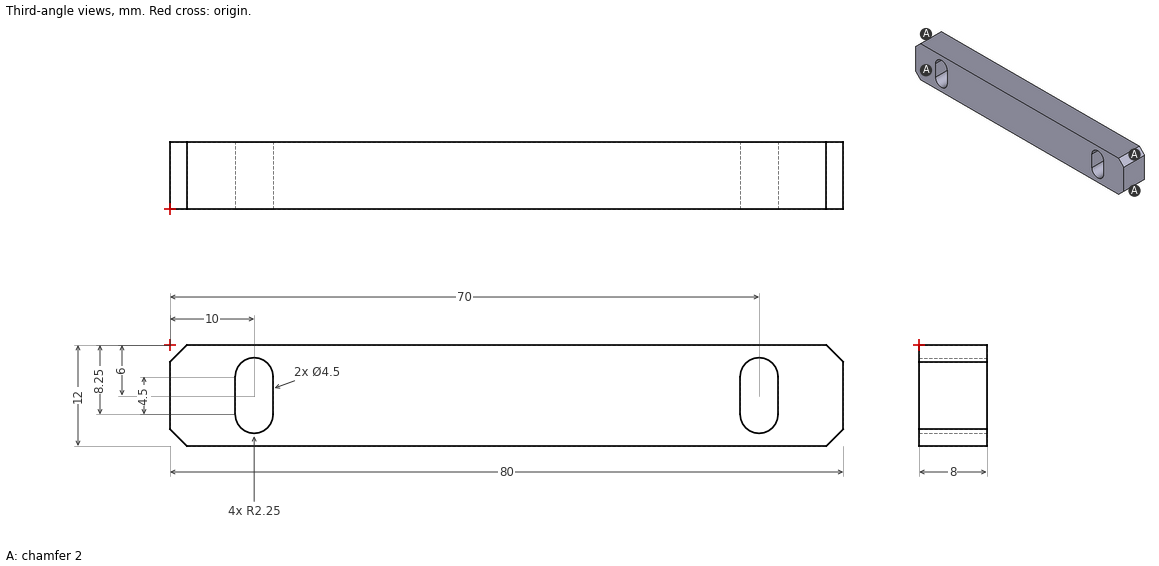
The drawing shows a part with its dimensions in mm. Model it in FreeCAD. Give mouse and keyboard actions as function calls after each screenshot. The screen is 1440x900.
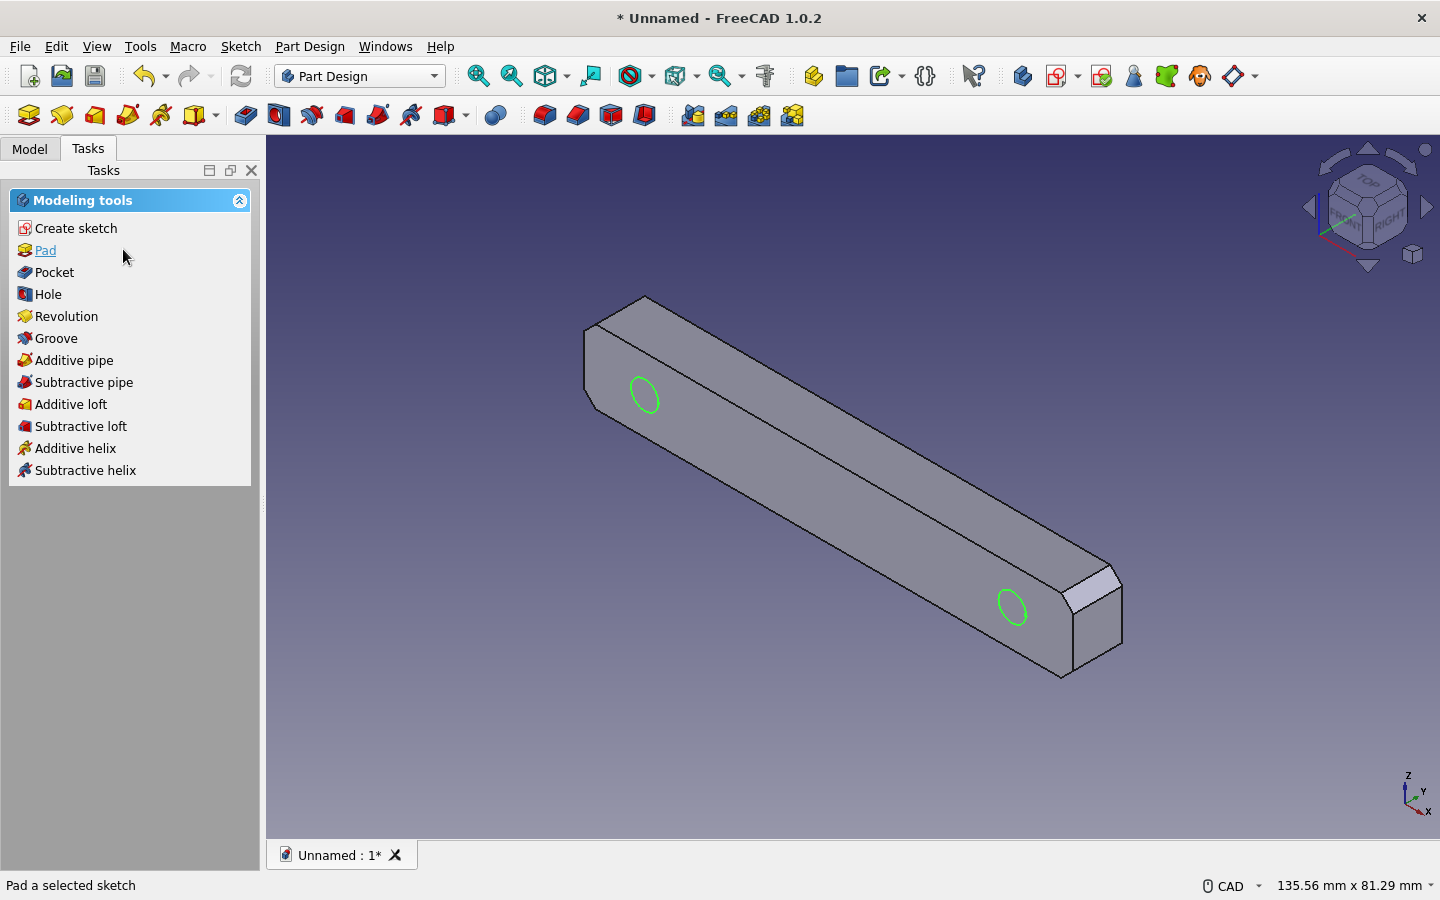
click(246, 116)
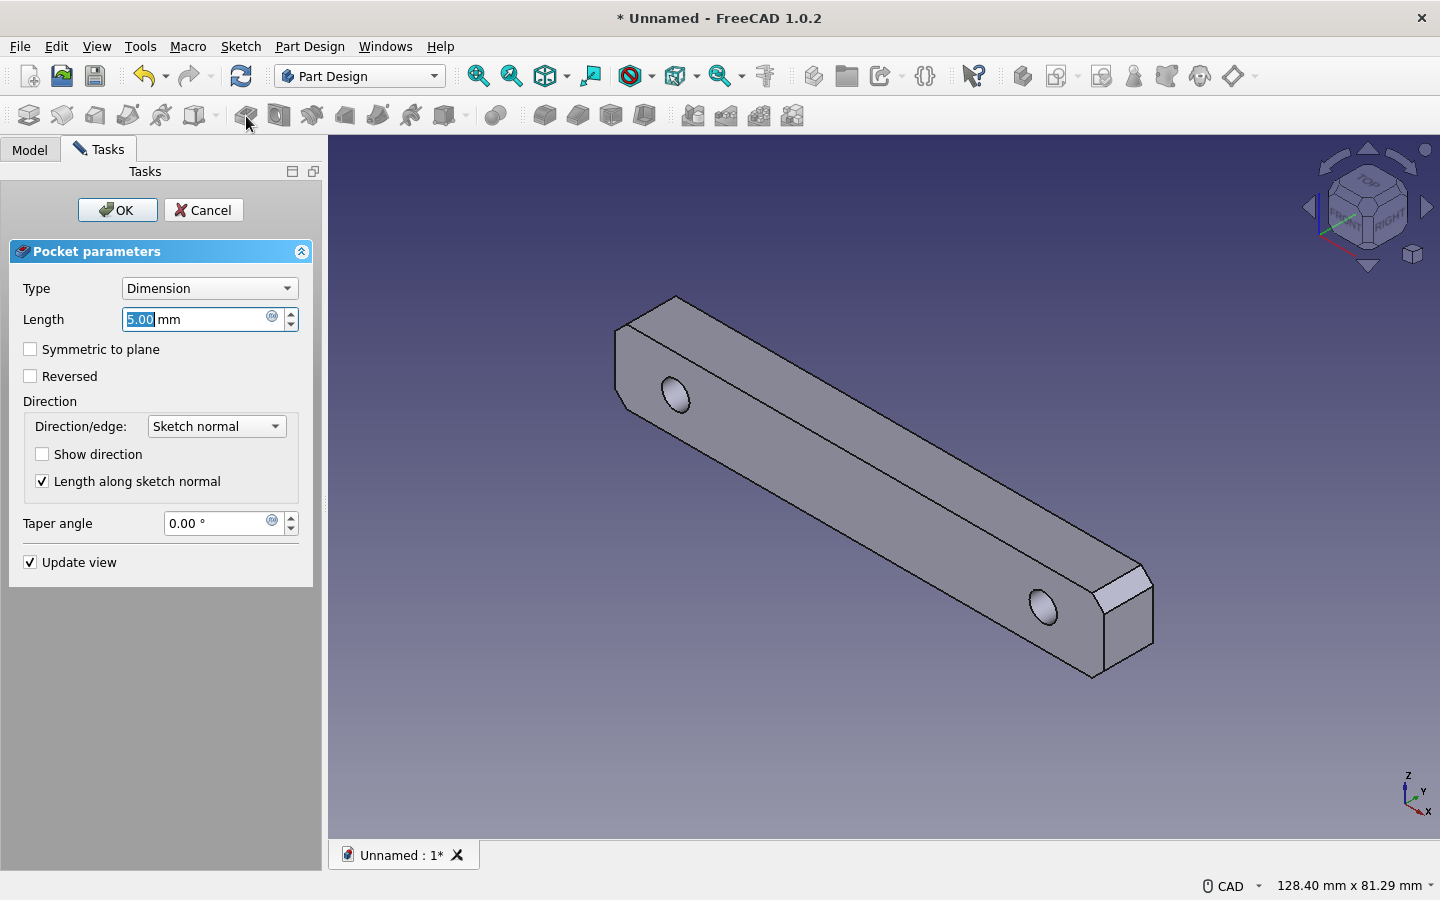
text(10)
key(Tab)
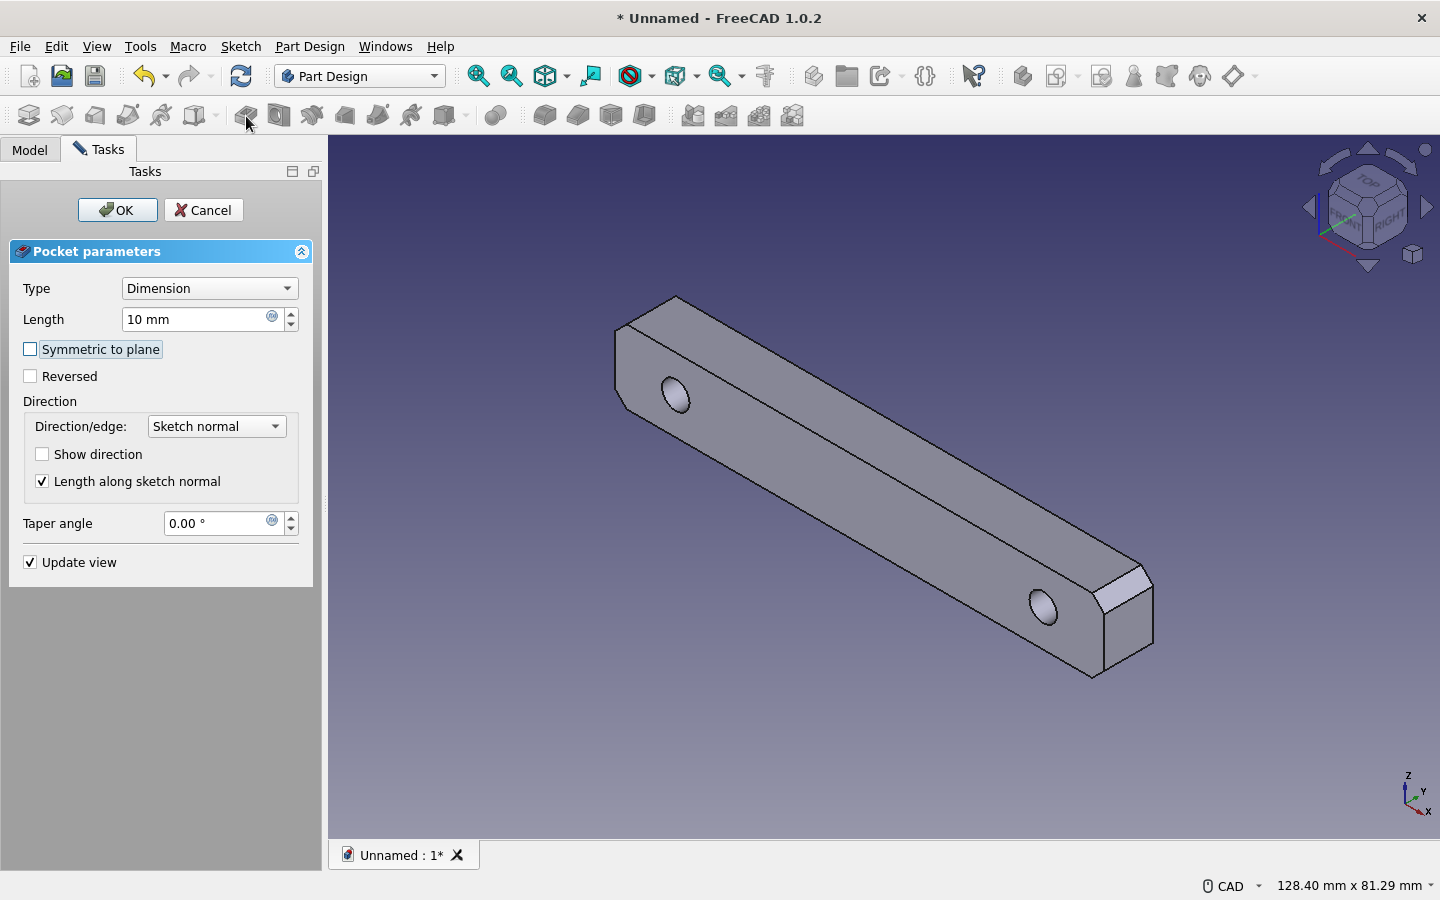
click(118, 210)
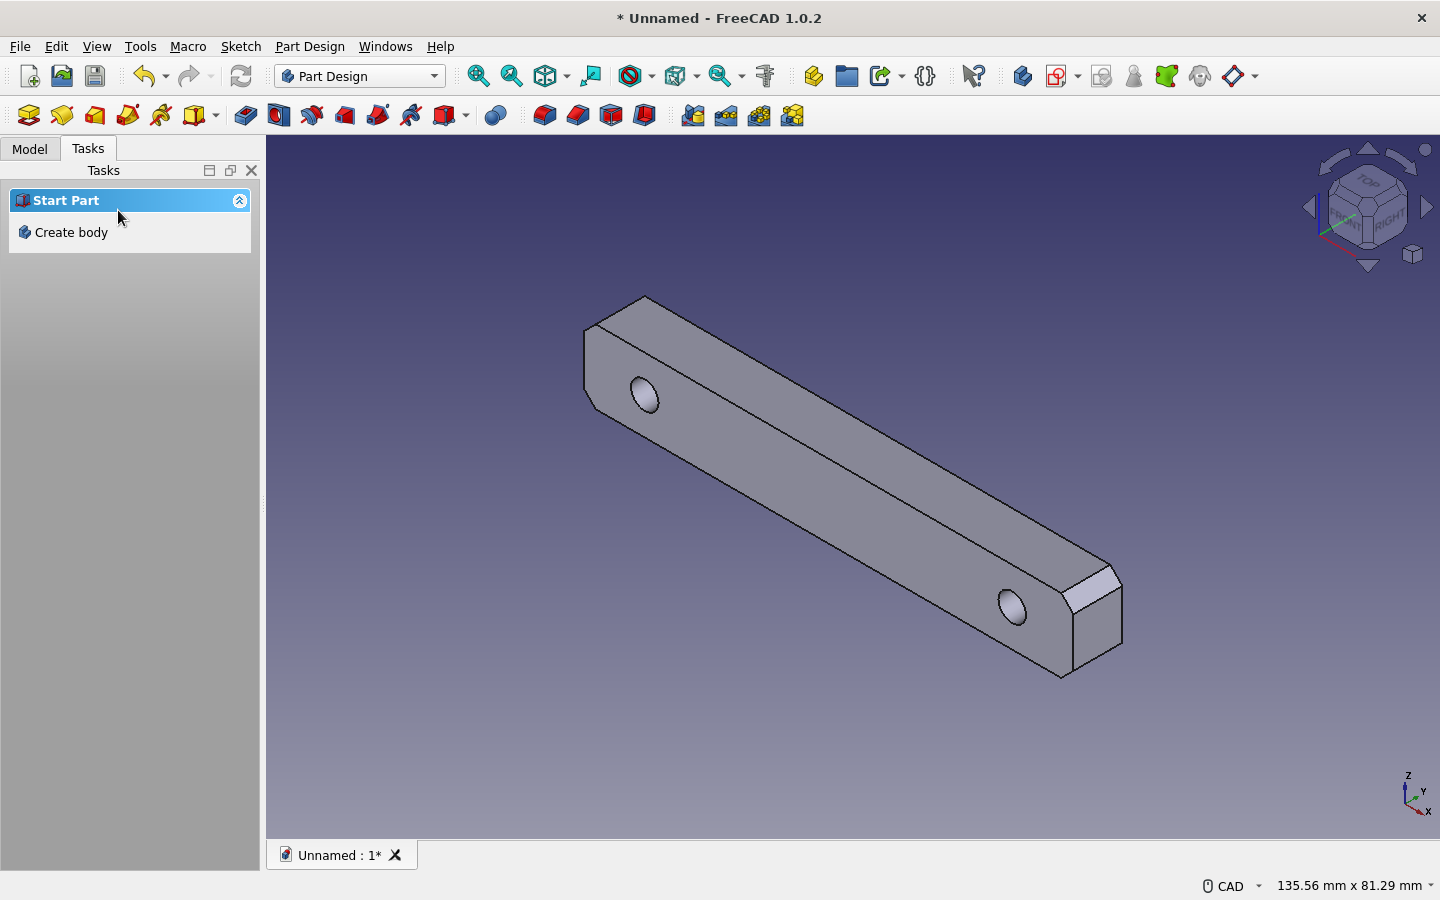
click(1056, 76)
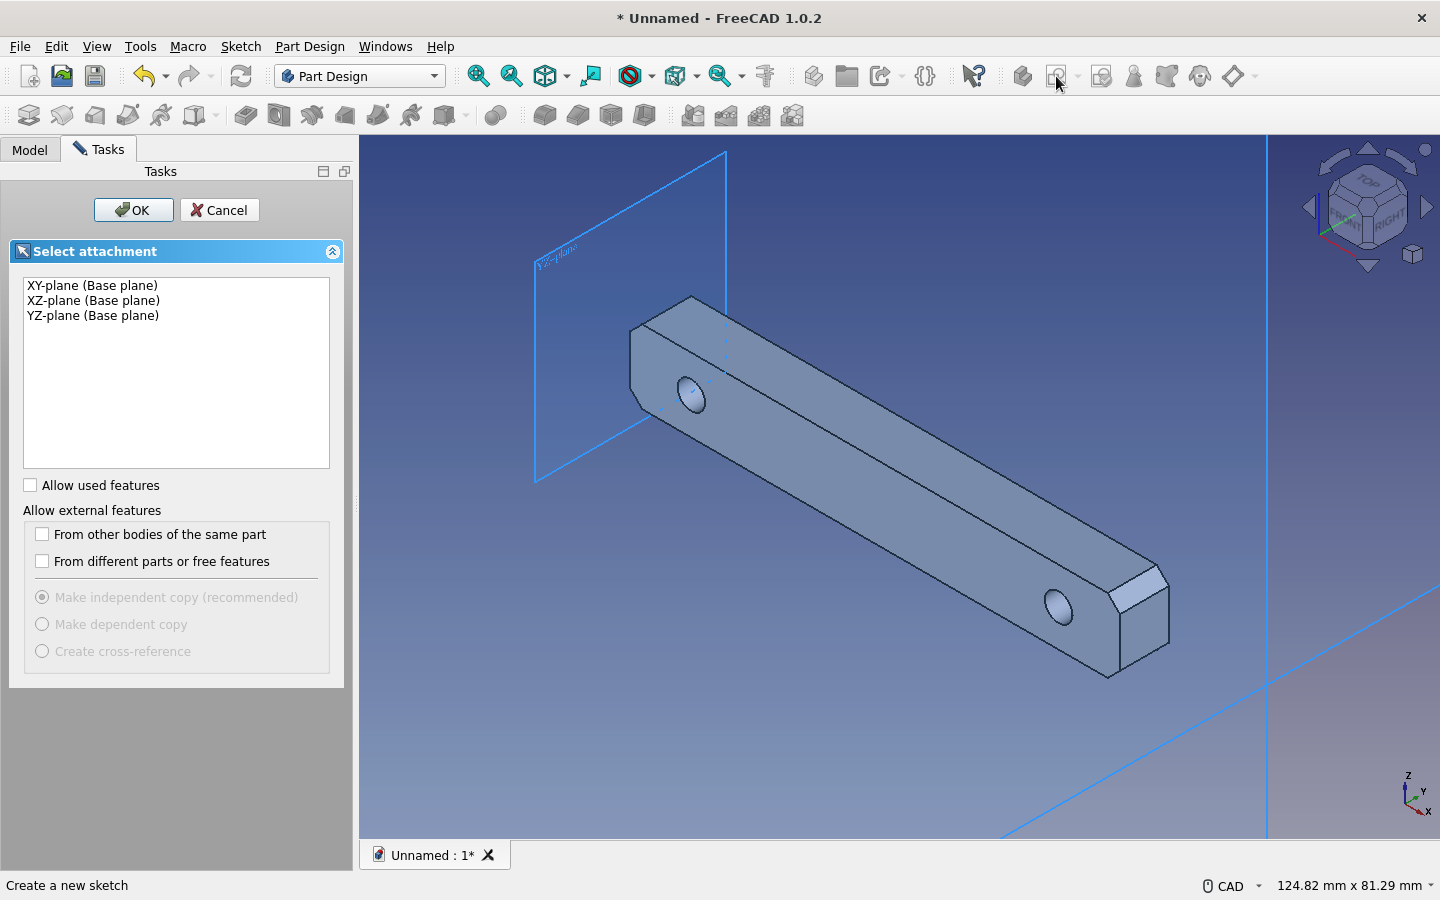
click(84, 300)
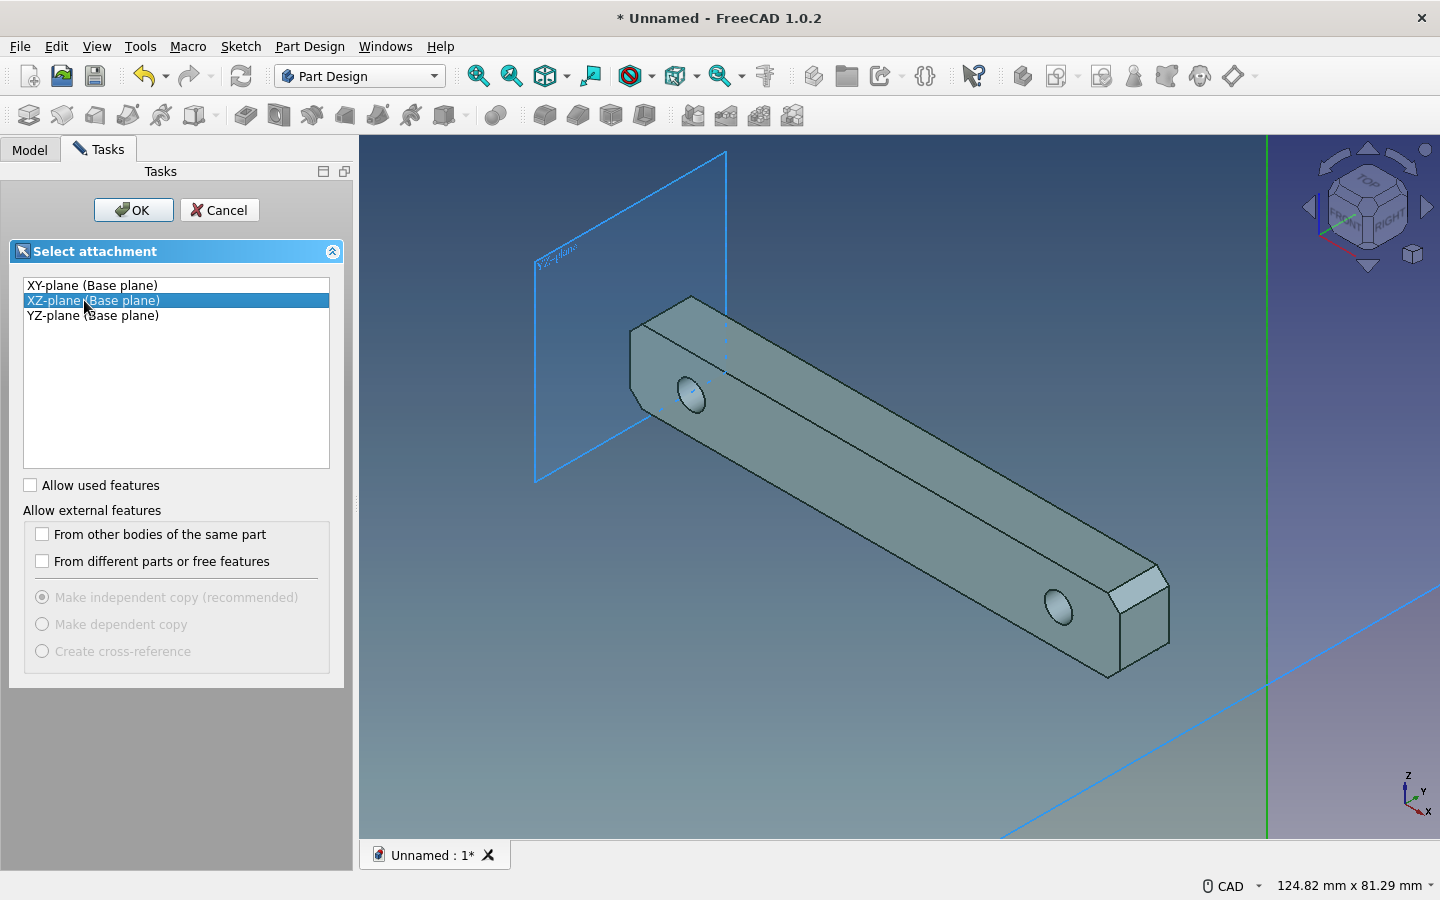
click(134, 210)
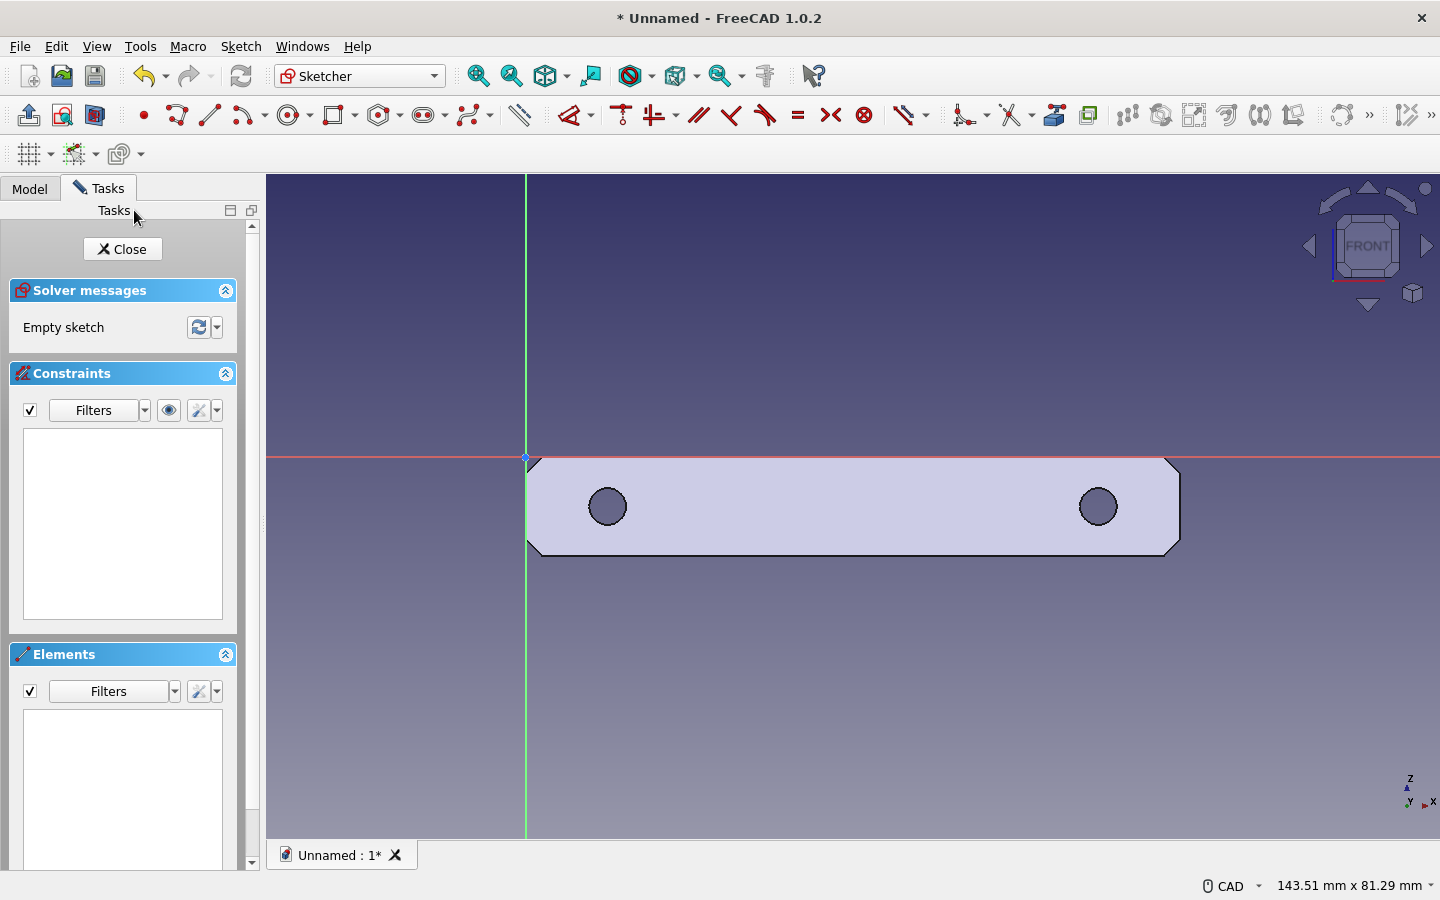
key(g)
key(s)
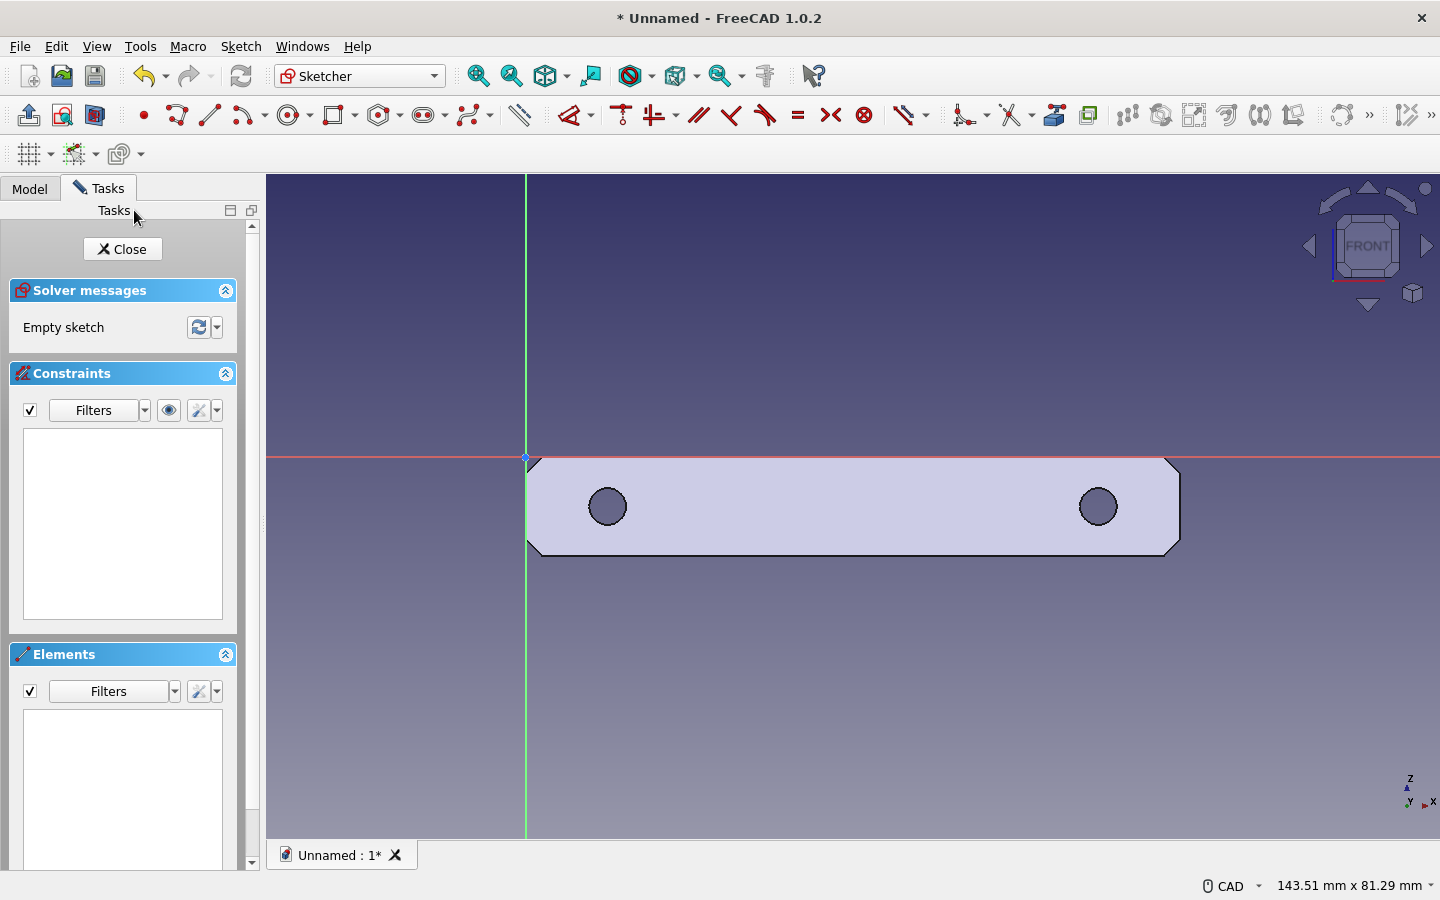
scroll(608, 525, up, 2)